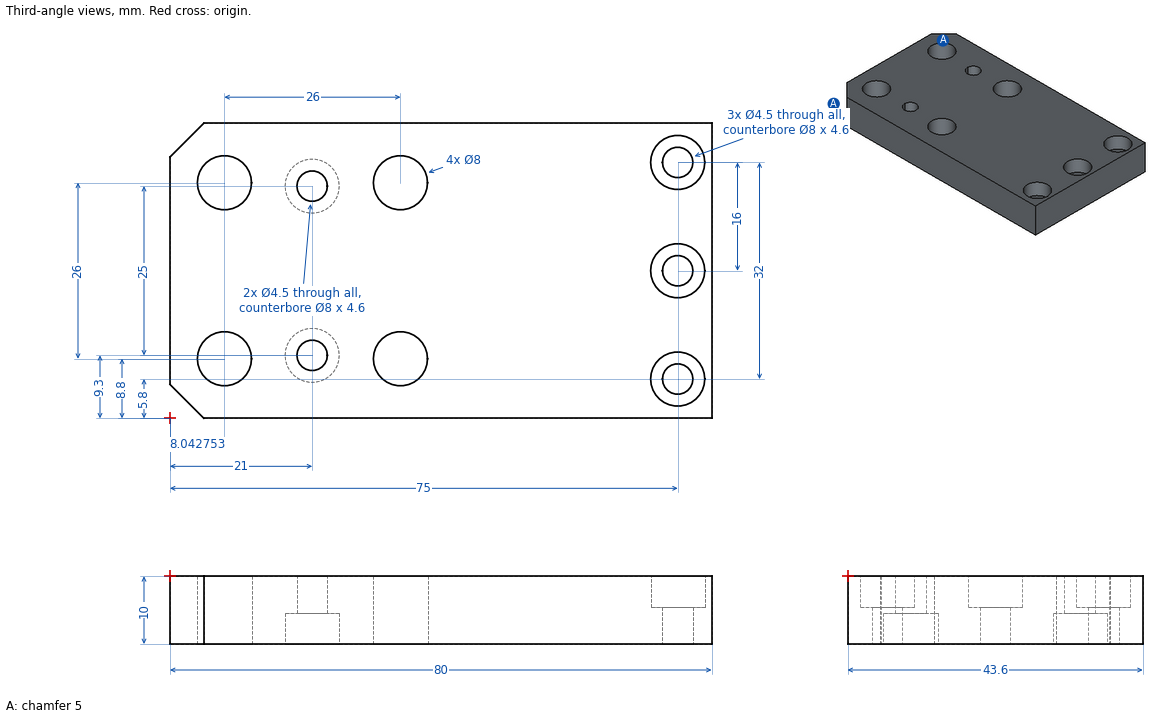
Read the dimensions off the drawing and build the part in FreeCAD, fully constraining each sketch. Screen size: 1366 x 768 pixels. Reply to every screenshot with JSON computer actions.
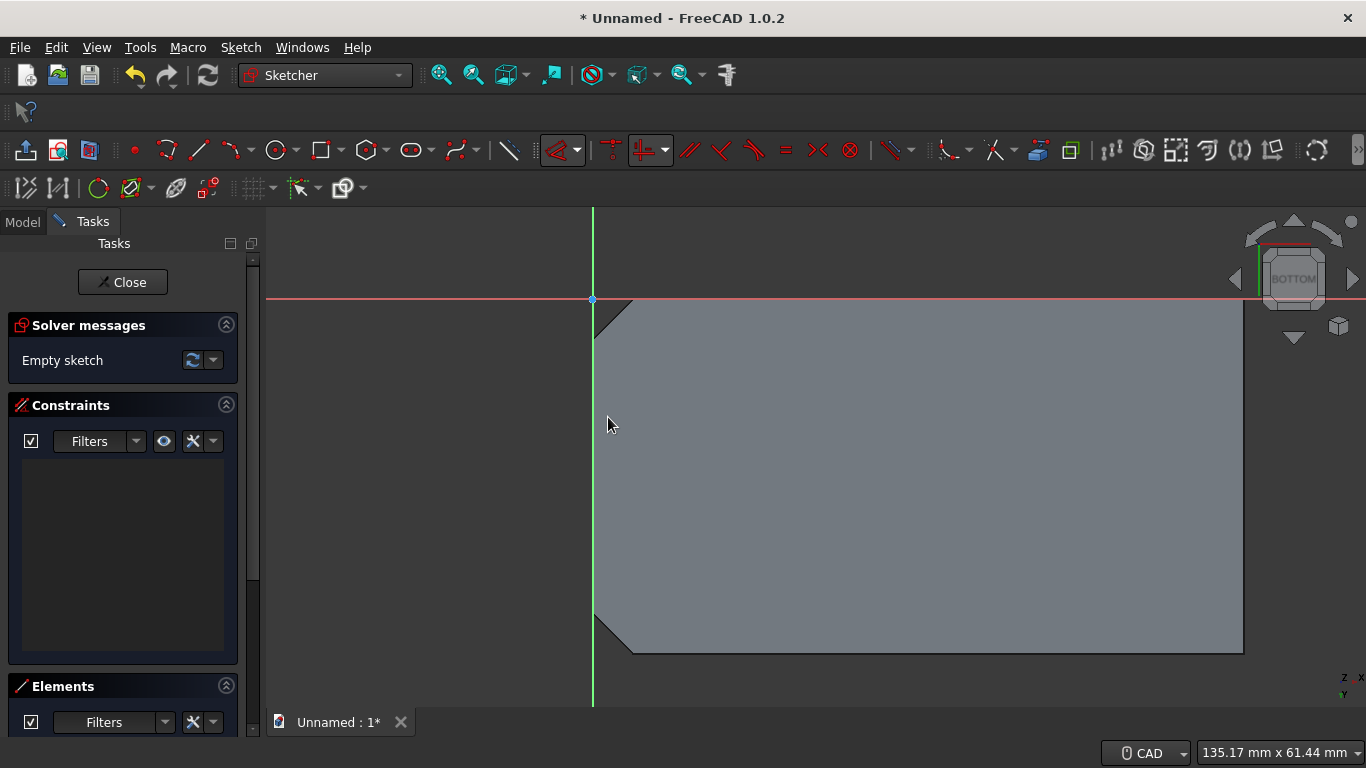
{"action": "left_click", "coordinate": [276, 150]}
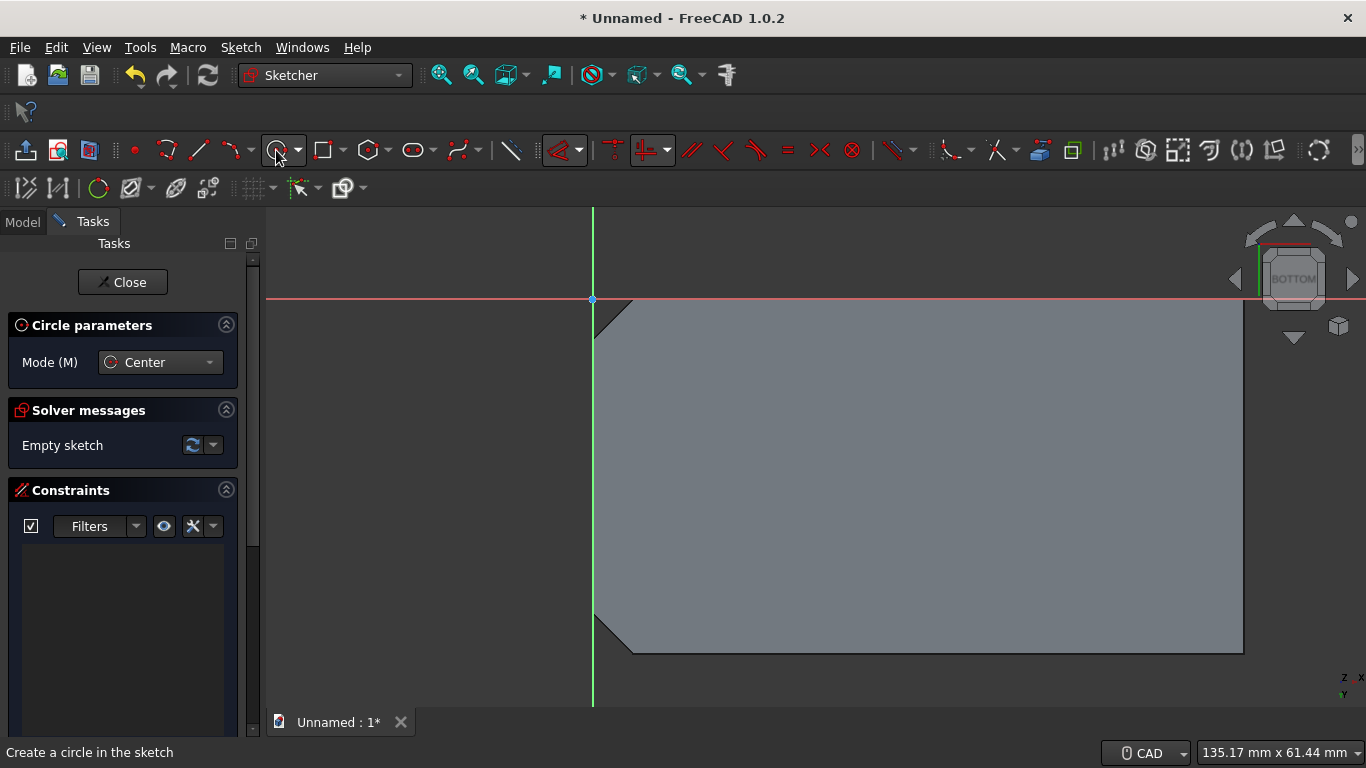
{"action": "left_click", "coordinate": [870, 582]}
{"action": "left_click", "coordinate": [893, 559]}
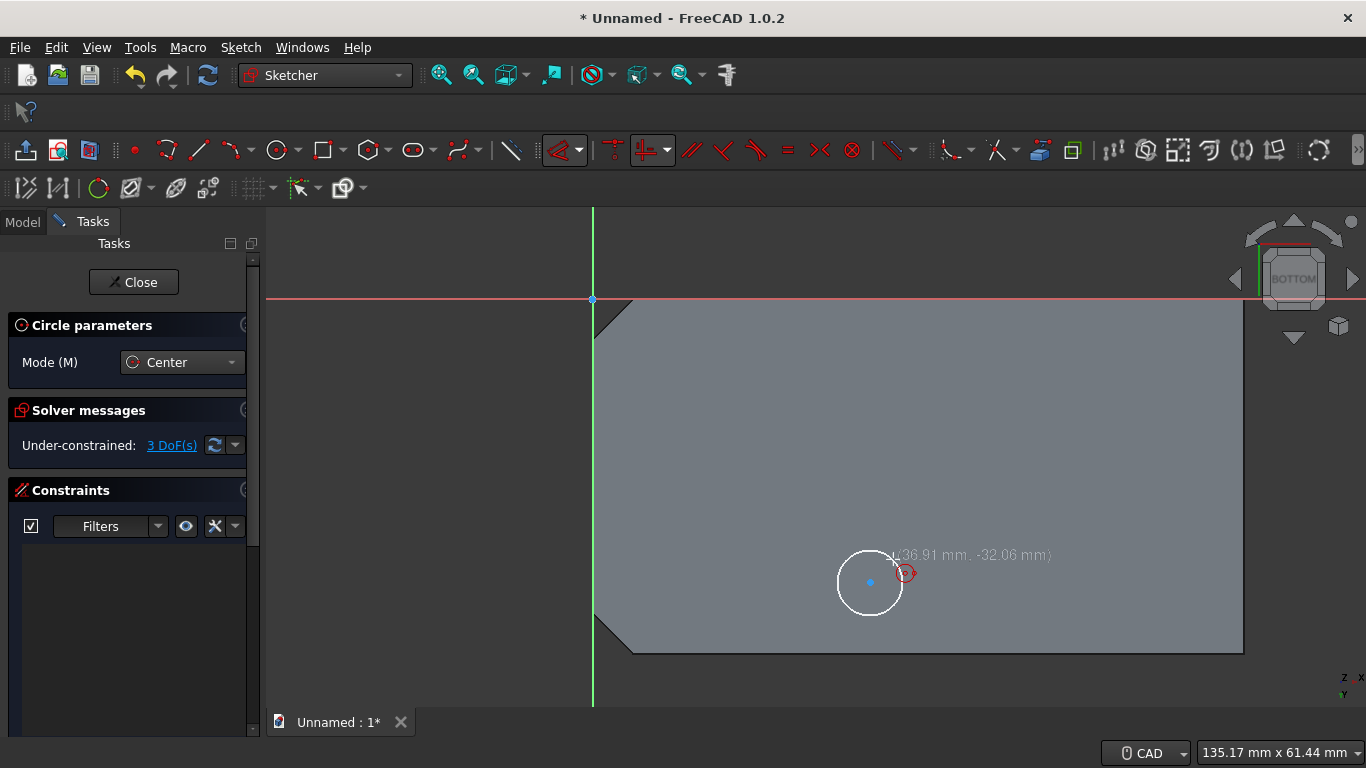
{"action": "left_click", "coordinate": [658, 582]}
{"action": "left_click", "coordinate": [681, 559]}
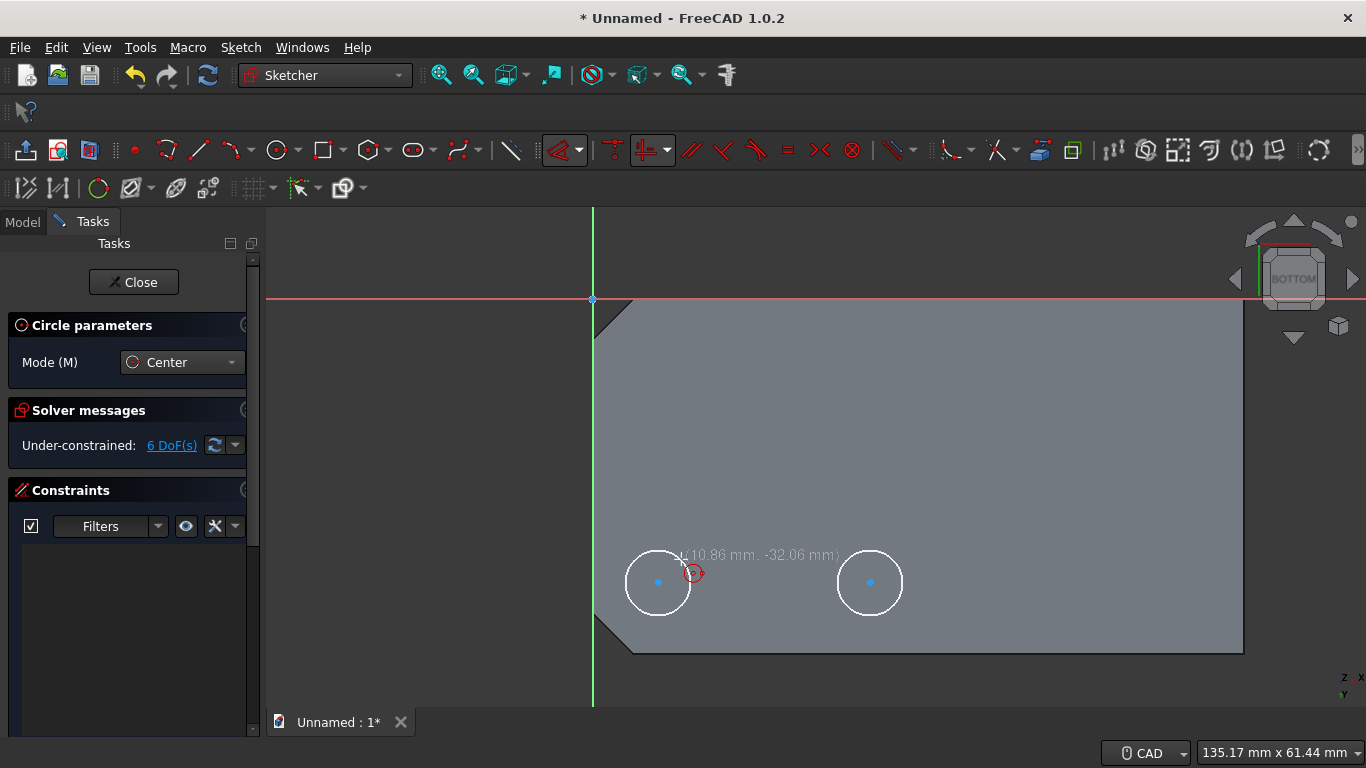
{"action": "left_click", "coordinate": [658, 371]}
{"action": "left_click", "coordinate": [681, 348]}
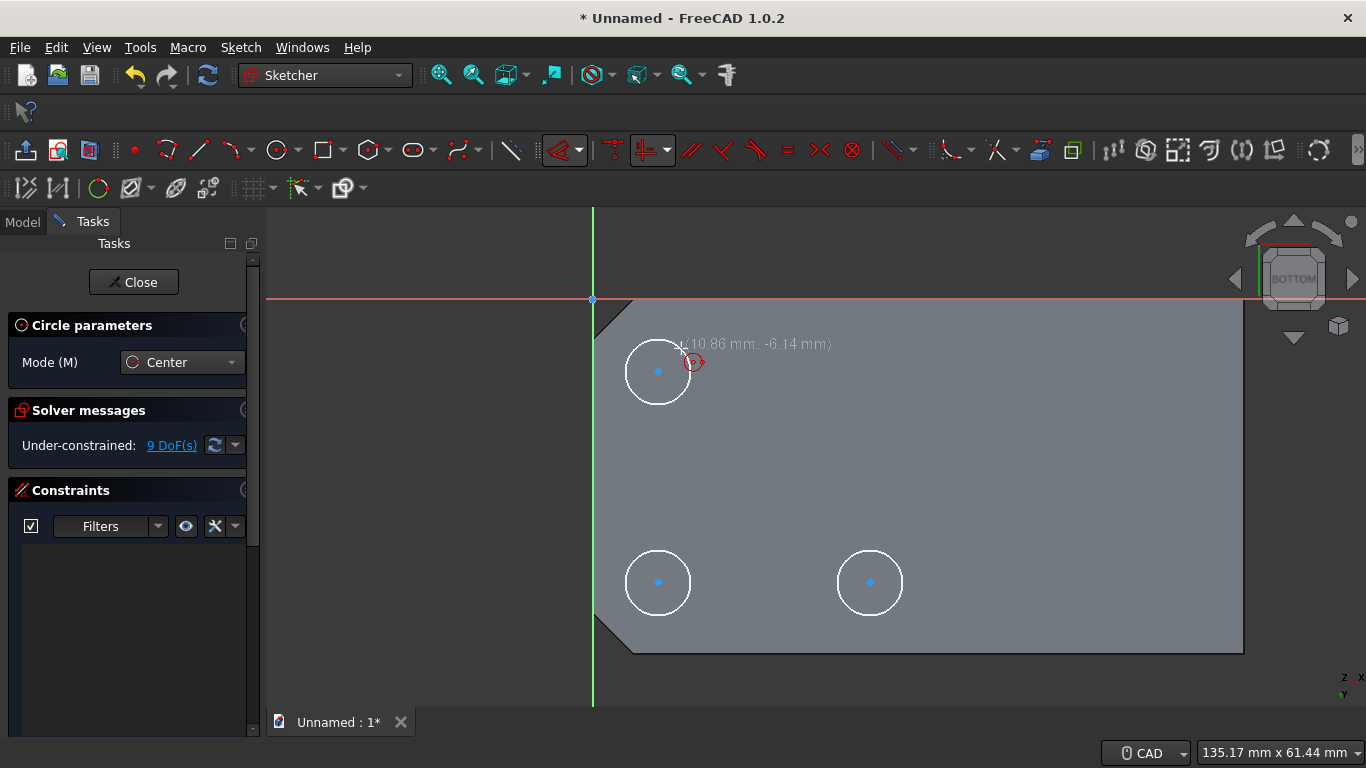
{"action": "left_click", "coordinate": [870, 371]}
{"action": "left_click", "coordinate": [893, 348]}
{"action": "key", "text": "Escape"}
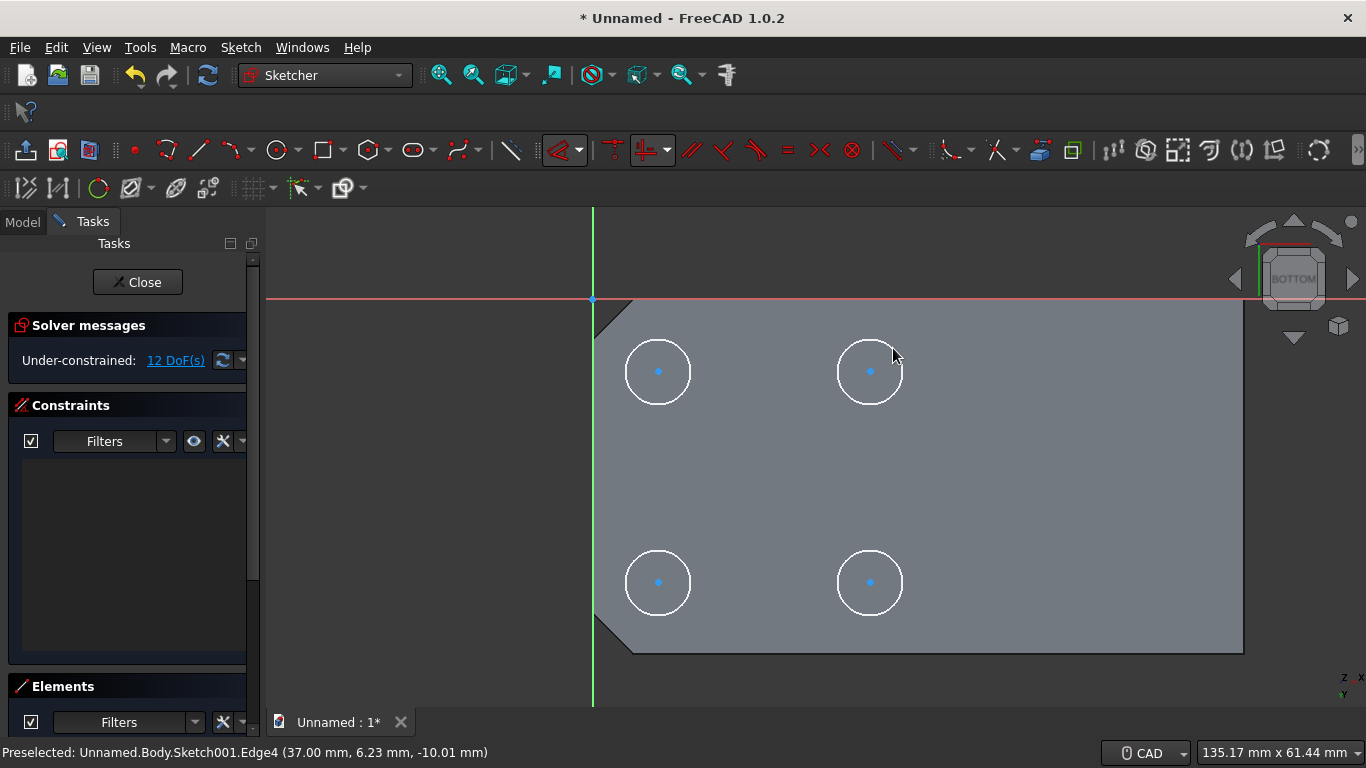
{"action": "left_click", "coordinate": [893, 560]}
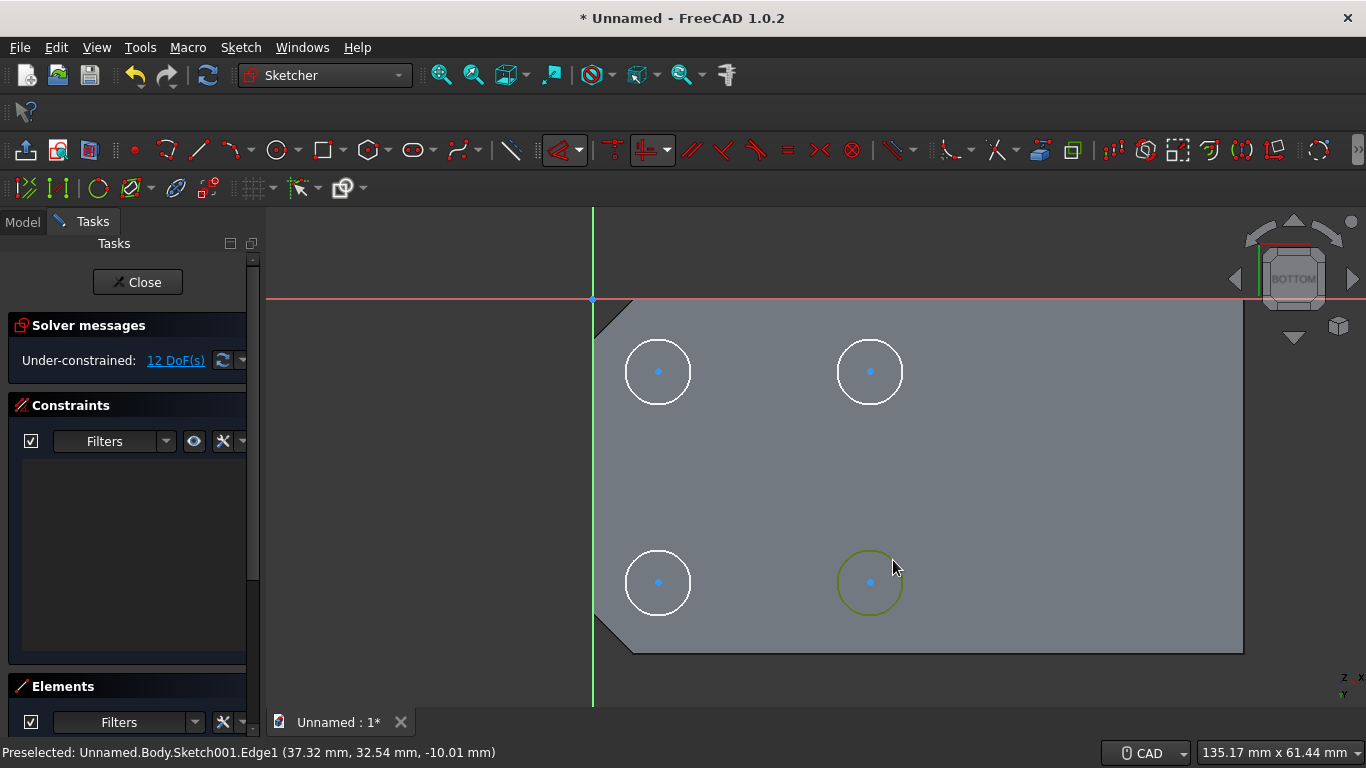
{"action": "left_click", "coordinate": [681, 560]}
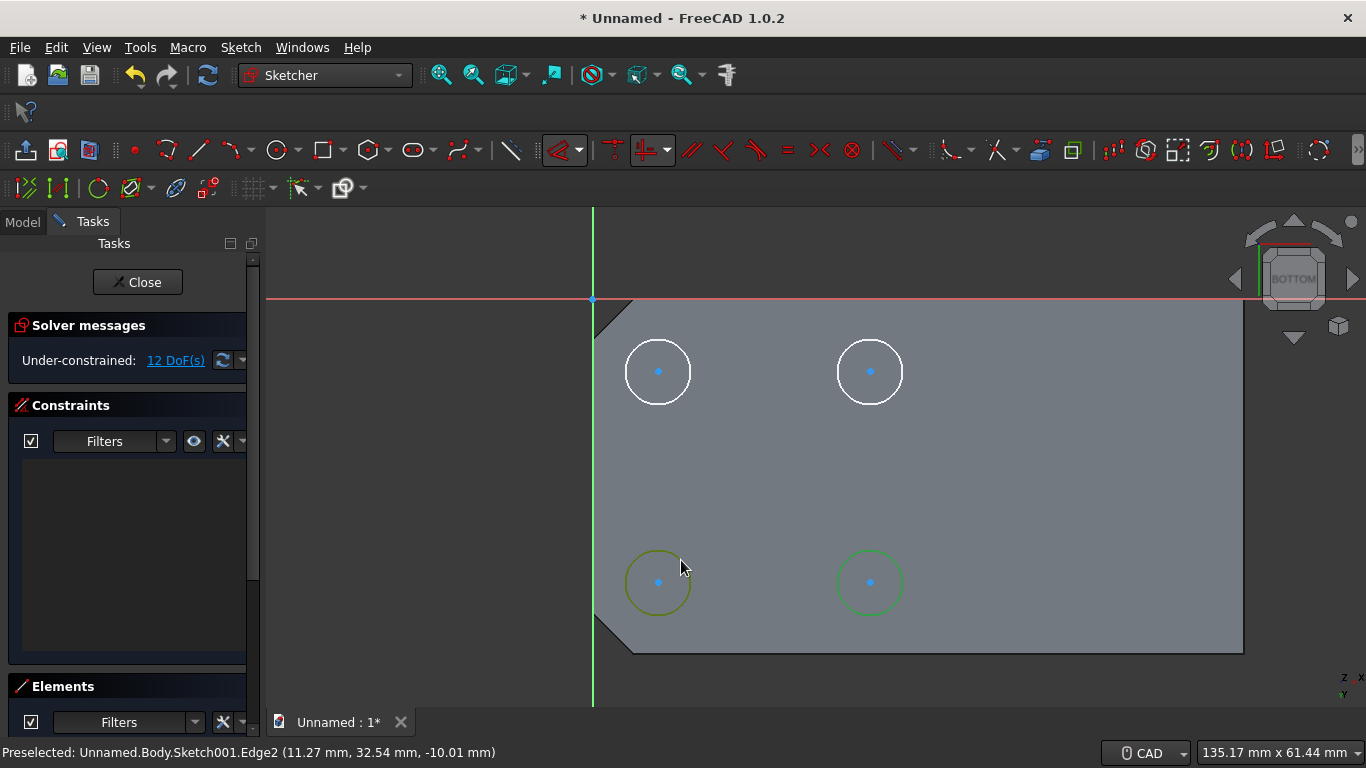
{"action": "left_click", "coordinate": [681, 349]}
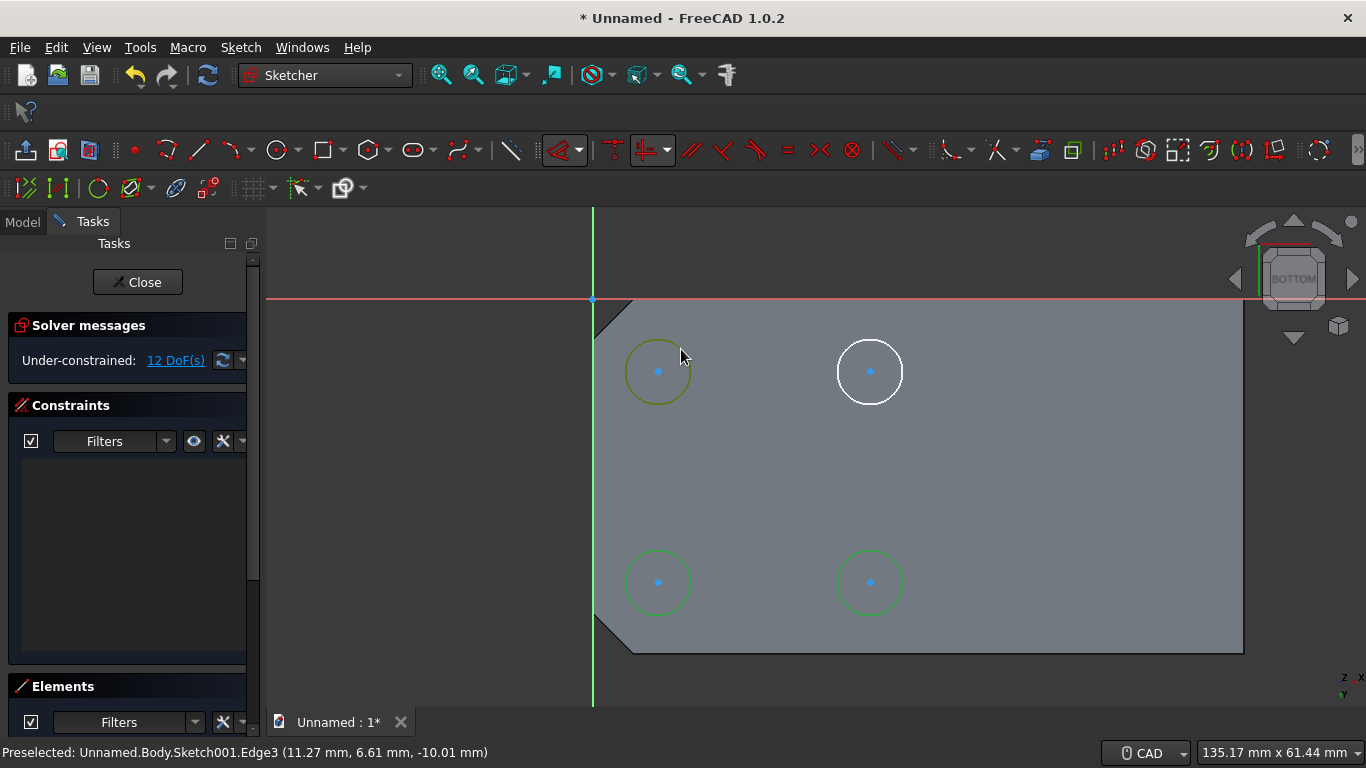
{"action": "left_click", "coordinate": [893, 349]}